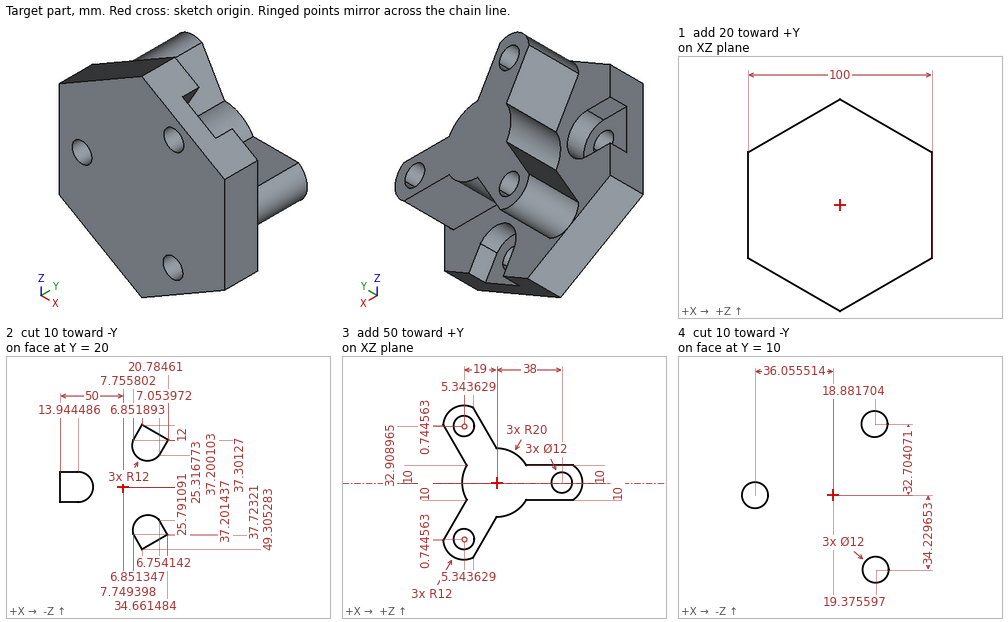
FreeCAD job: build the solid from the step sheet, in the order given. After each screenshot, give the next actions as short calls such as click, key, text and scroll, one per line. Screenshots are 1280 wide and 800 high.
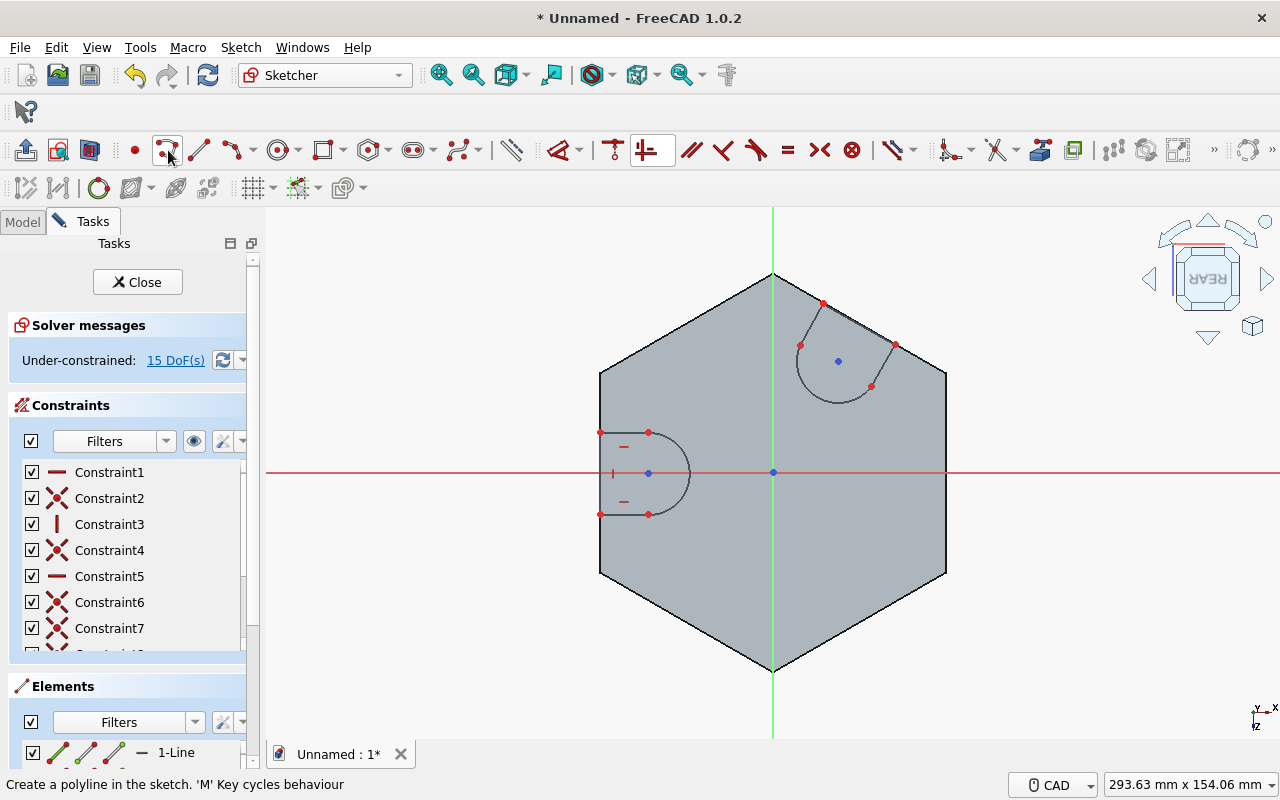
click(800, 601)
click(823, 643)
click(893, 603)
click(869, 562)
right_click(869, 562)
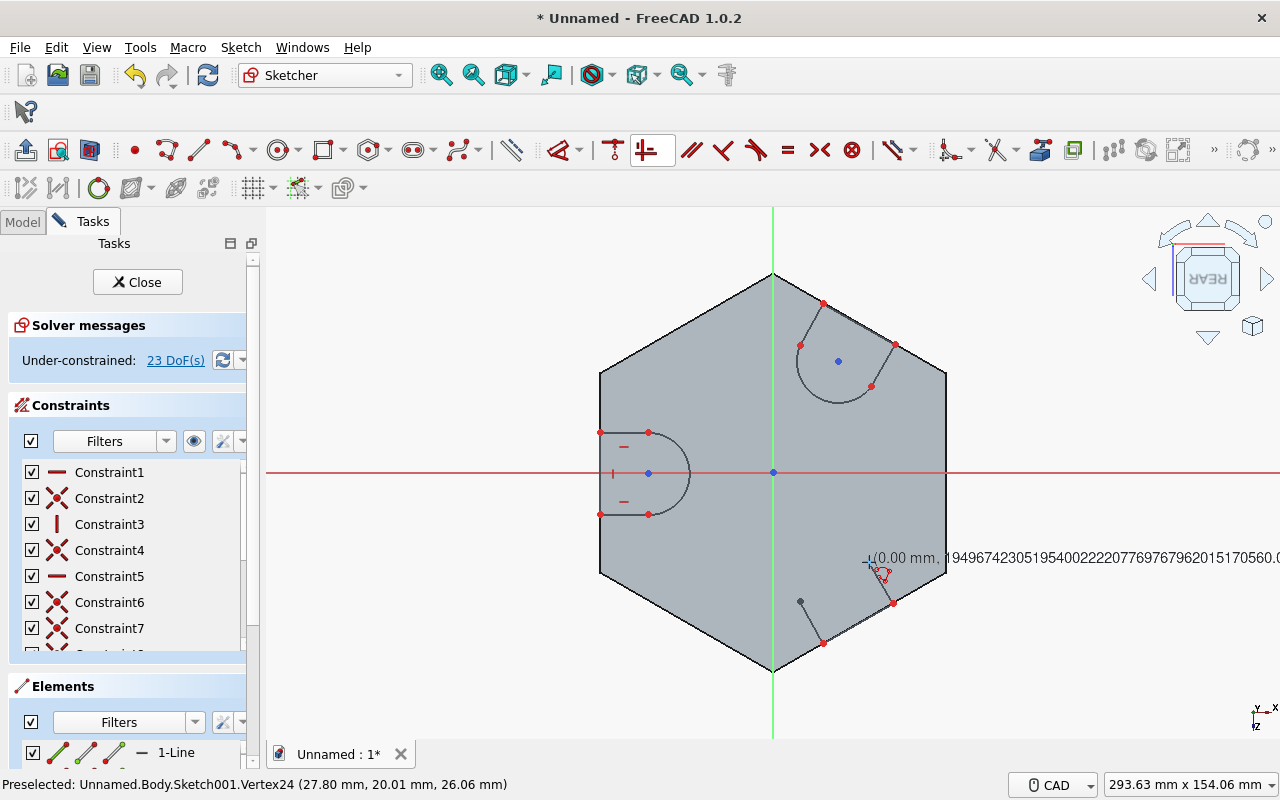
key(g)
key(3)
key(a)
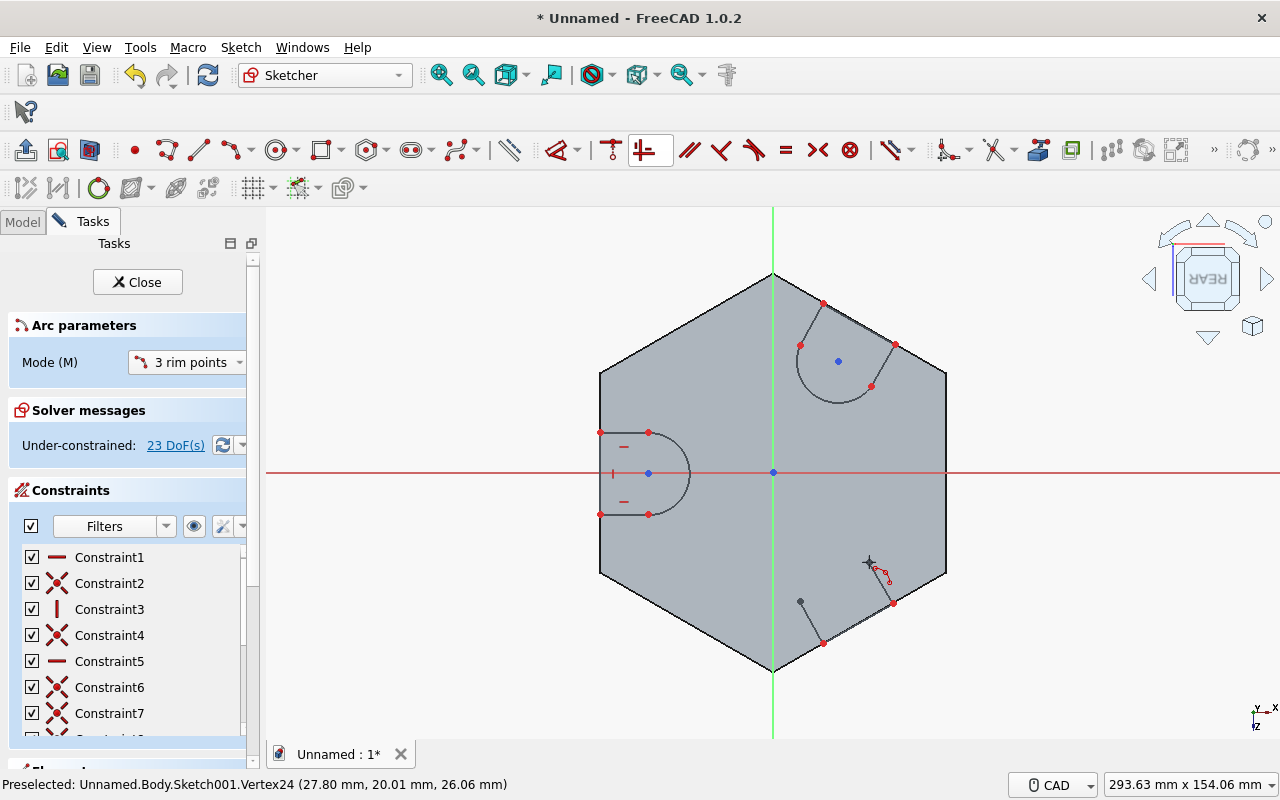
click(869, 563)
click(800, 602)
click(819, 555)
key(Escape)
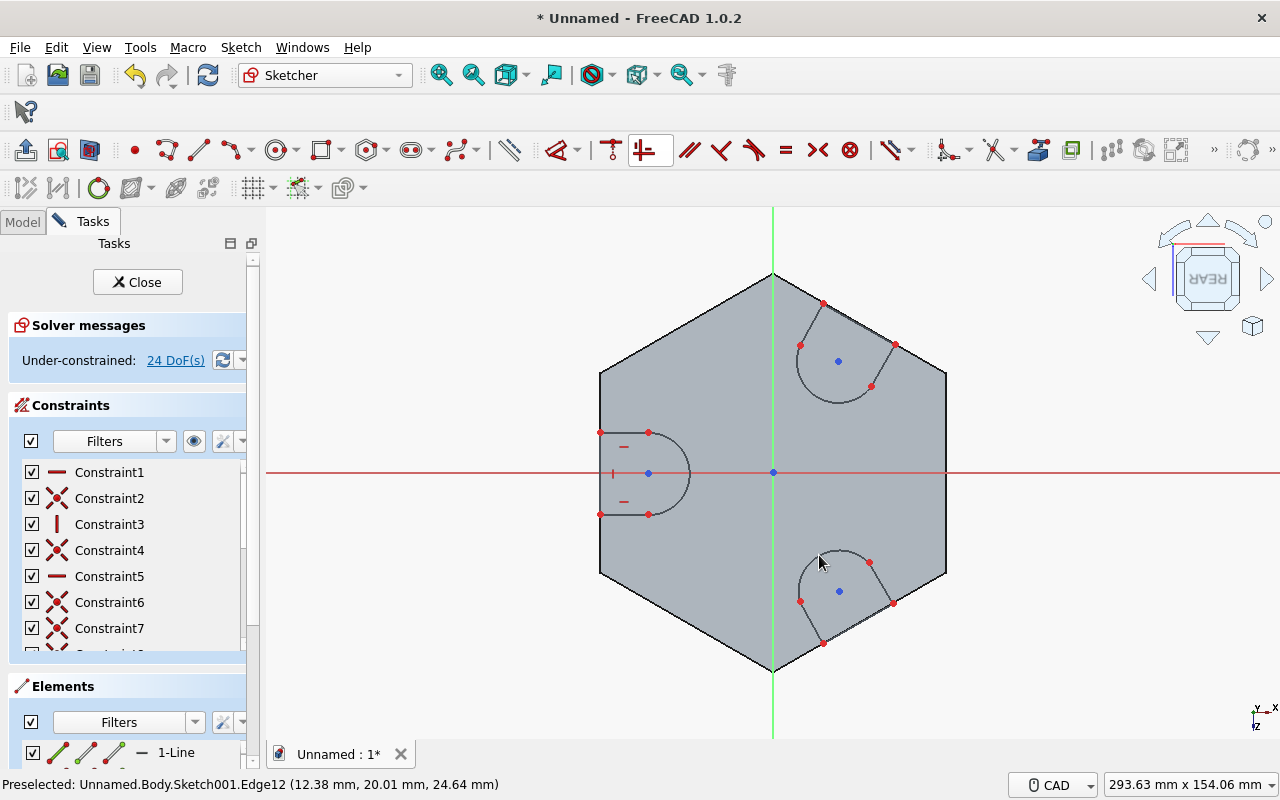
click(634, 433)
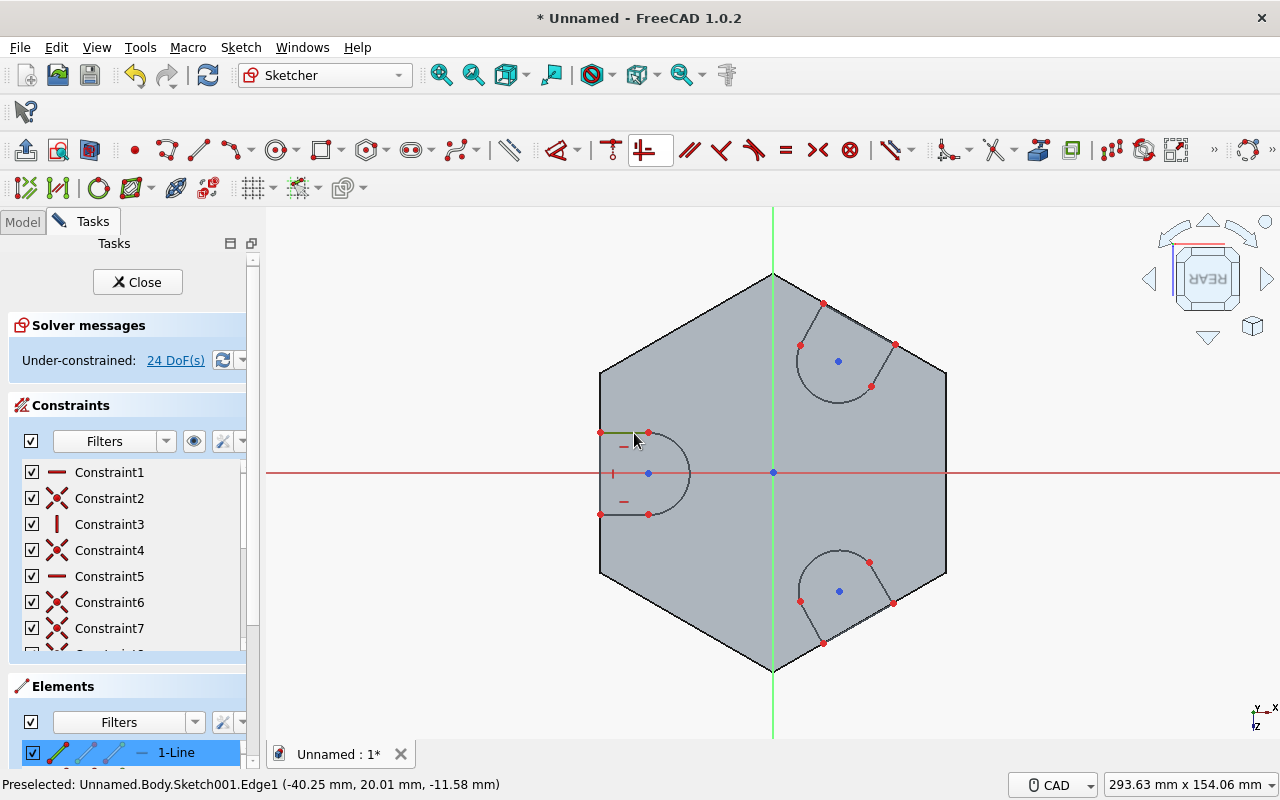
click(682, 498)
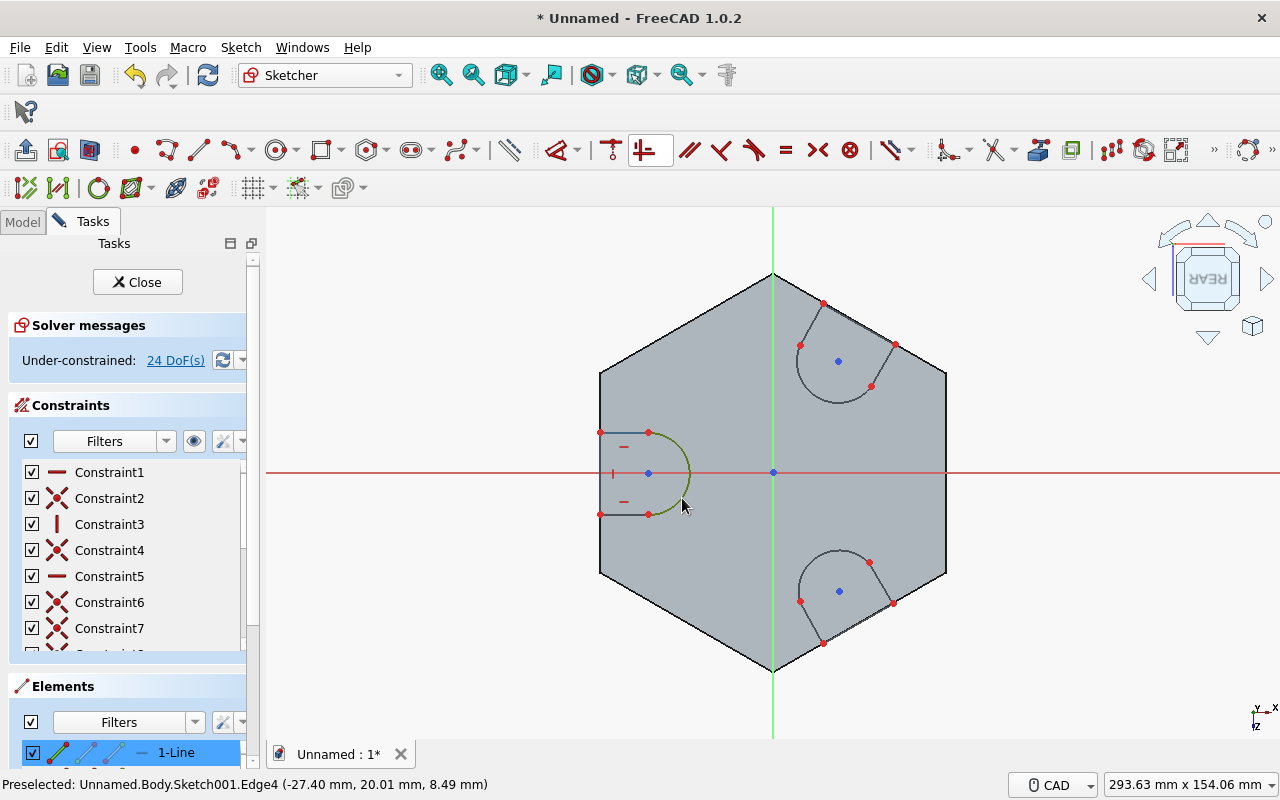
click(754, 150)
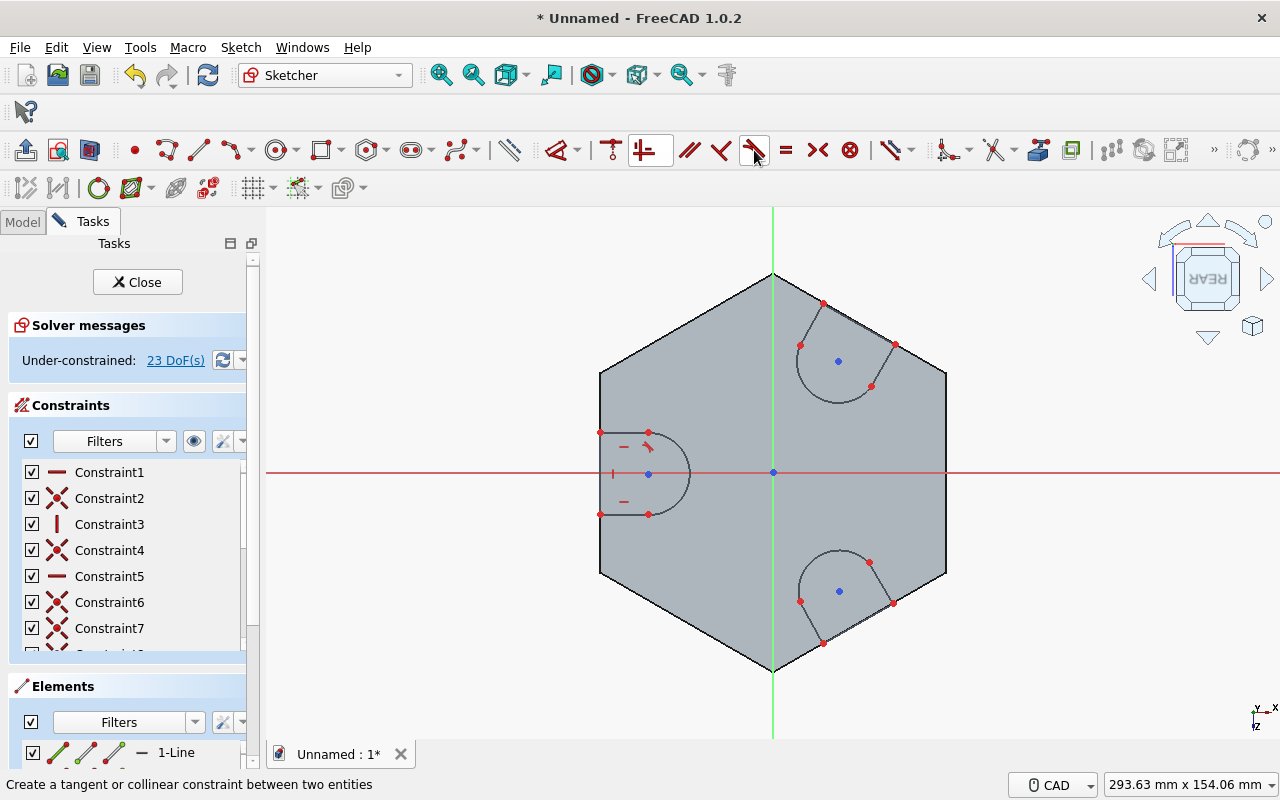
click(614, 515)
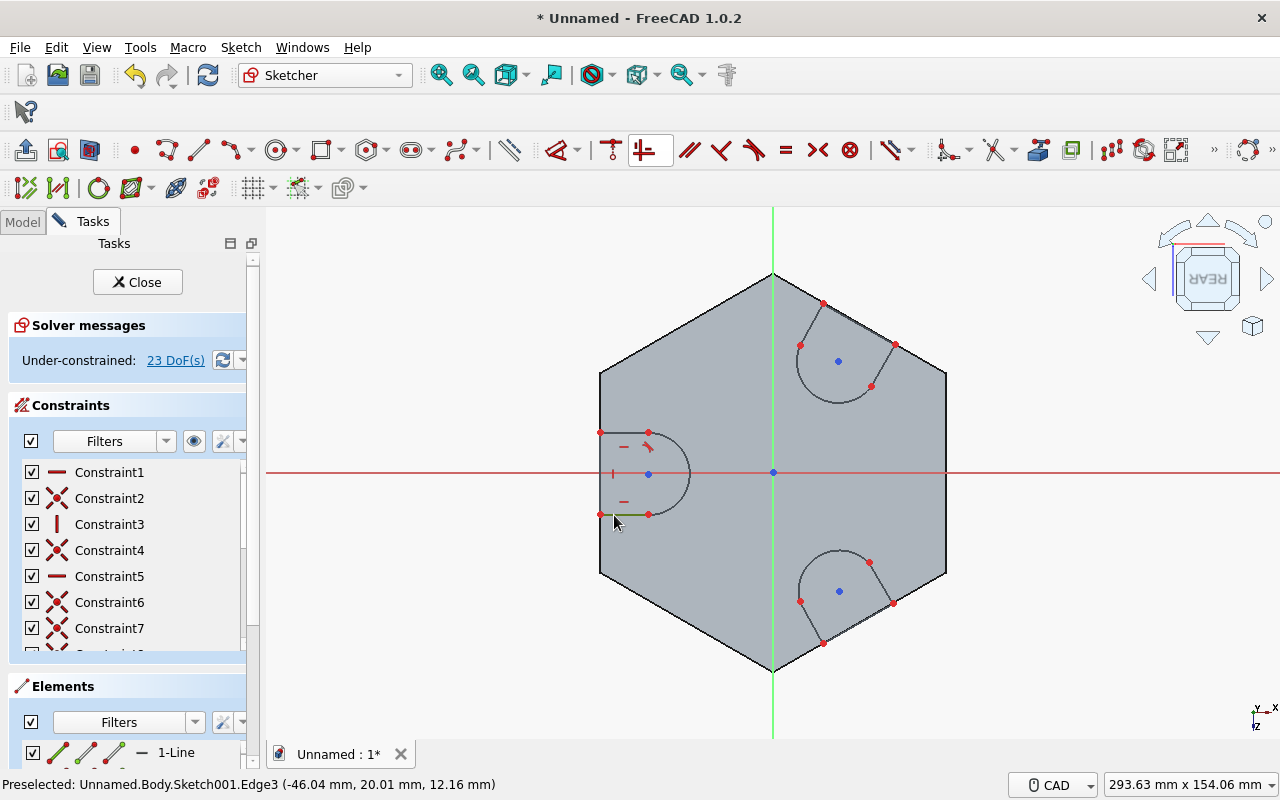
click(682, 499)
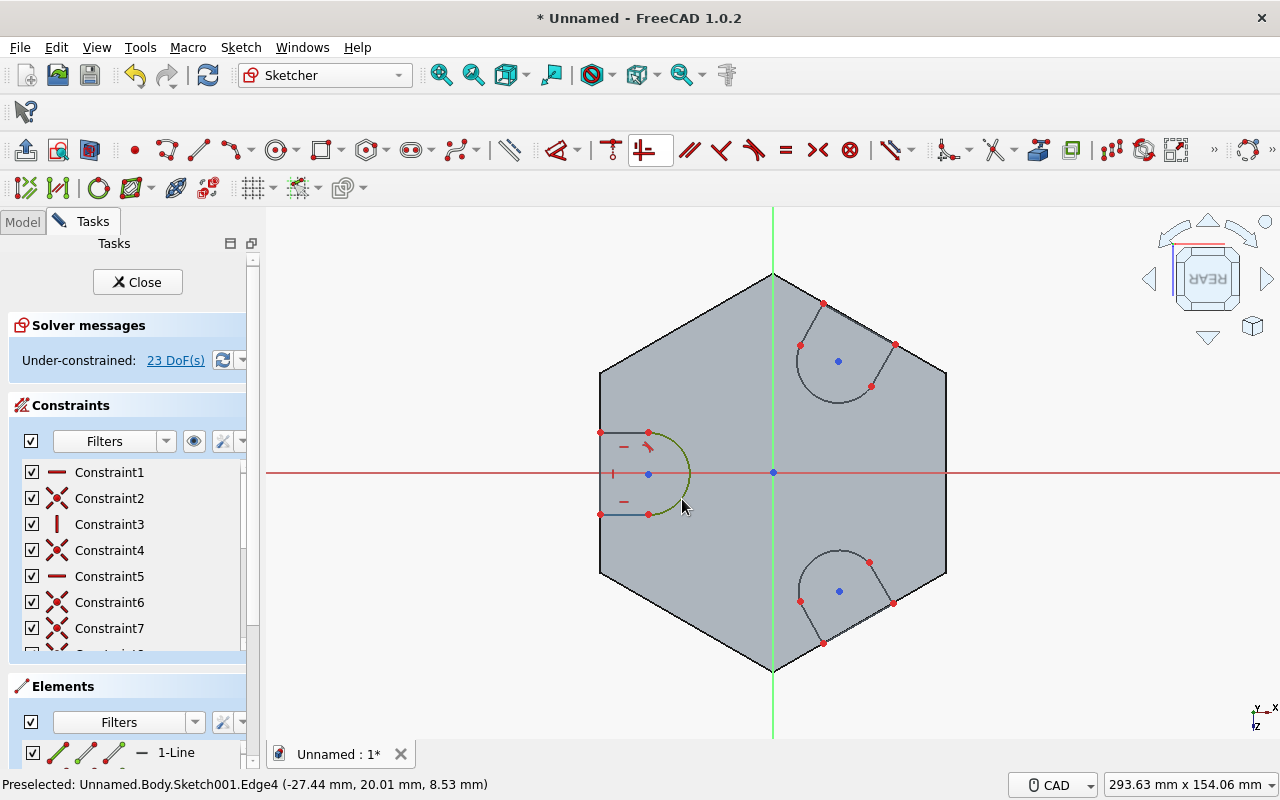
click(754, 150)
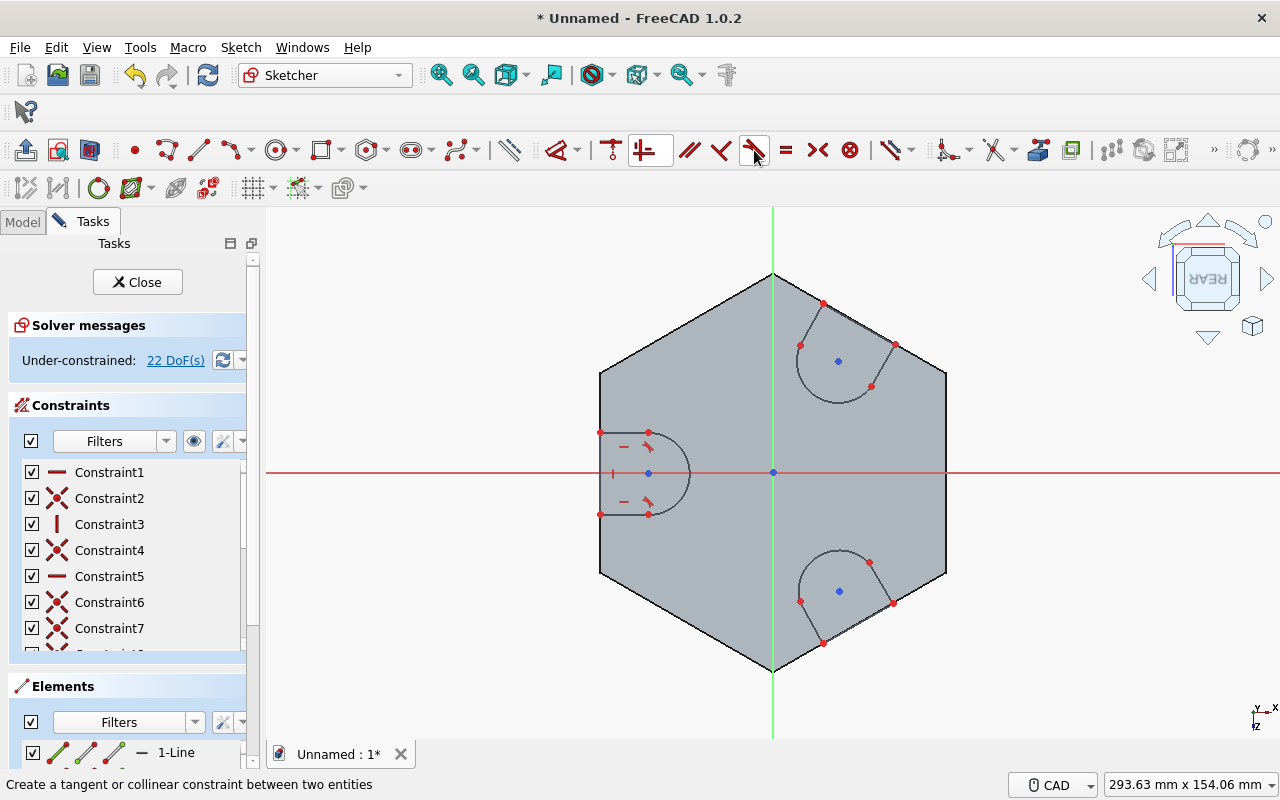
click(682, 498)